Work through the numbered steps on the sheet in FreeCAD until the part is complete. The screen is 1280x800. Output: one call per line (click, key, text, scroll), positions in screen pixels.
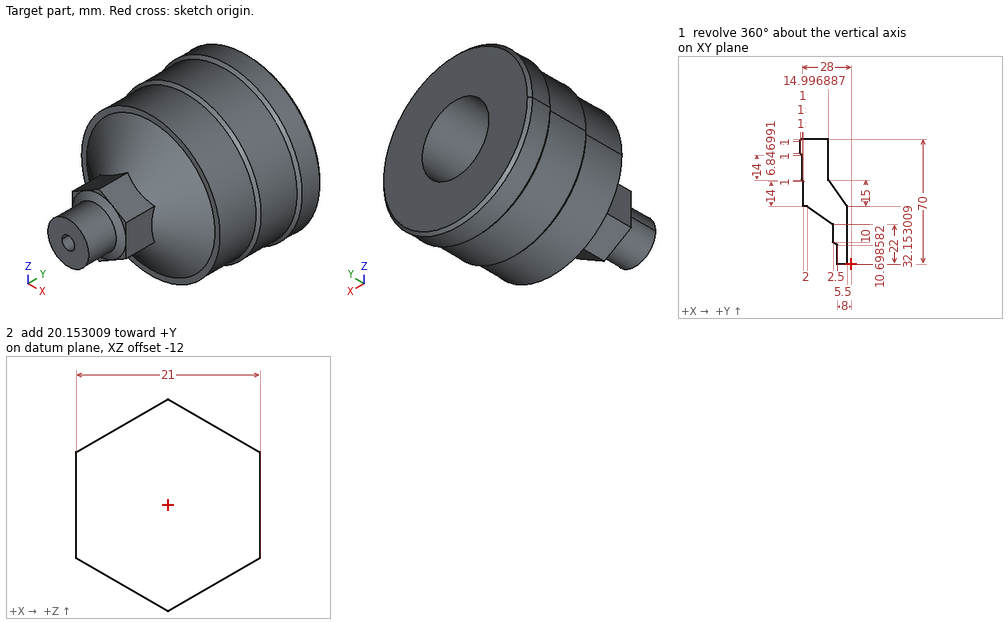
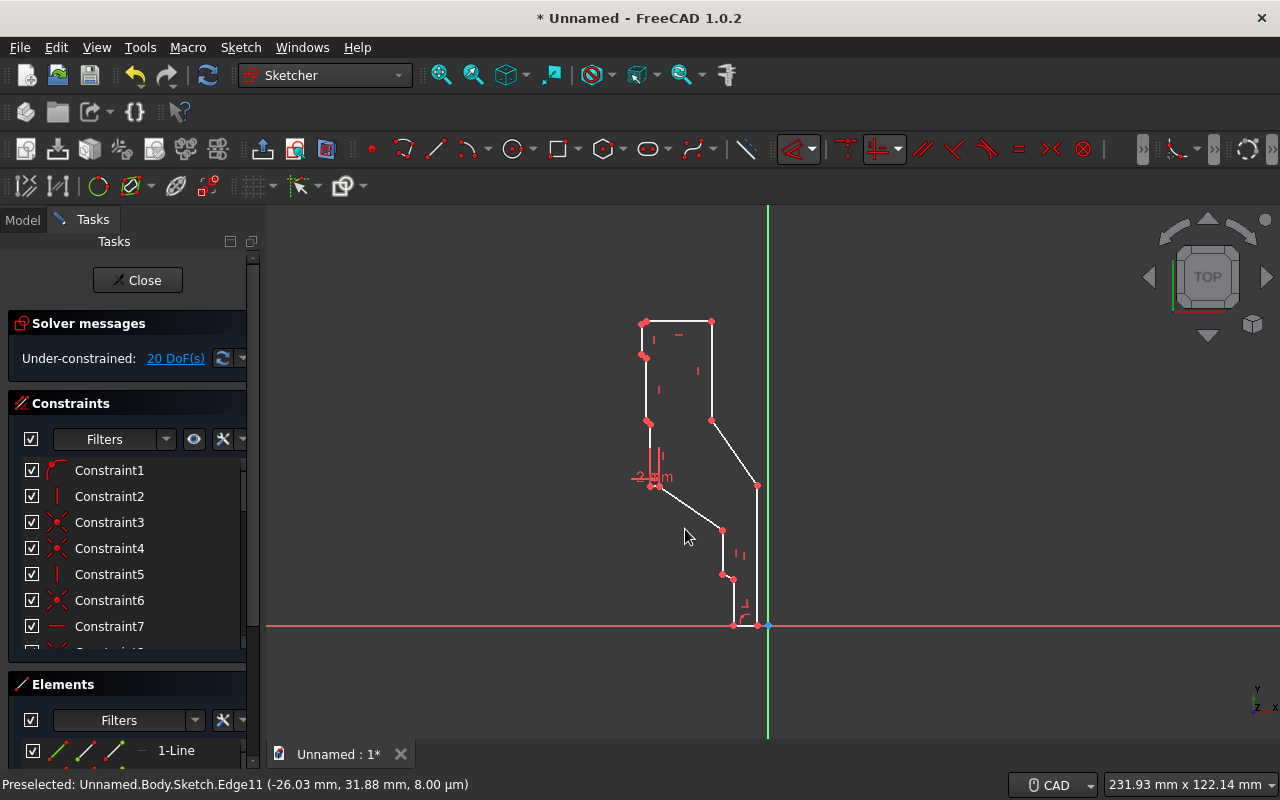
click(646, 377)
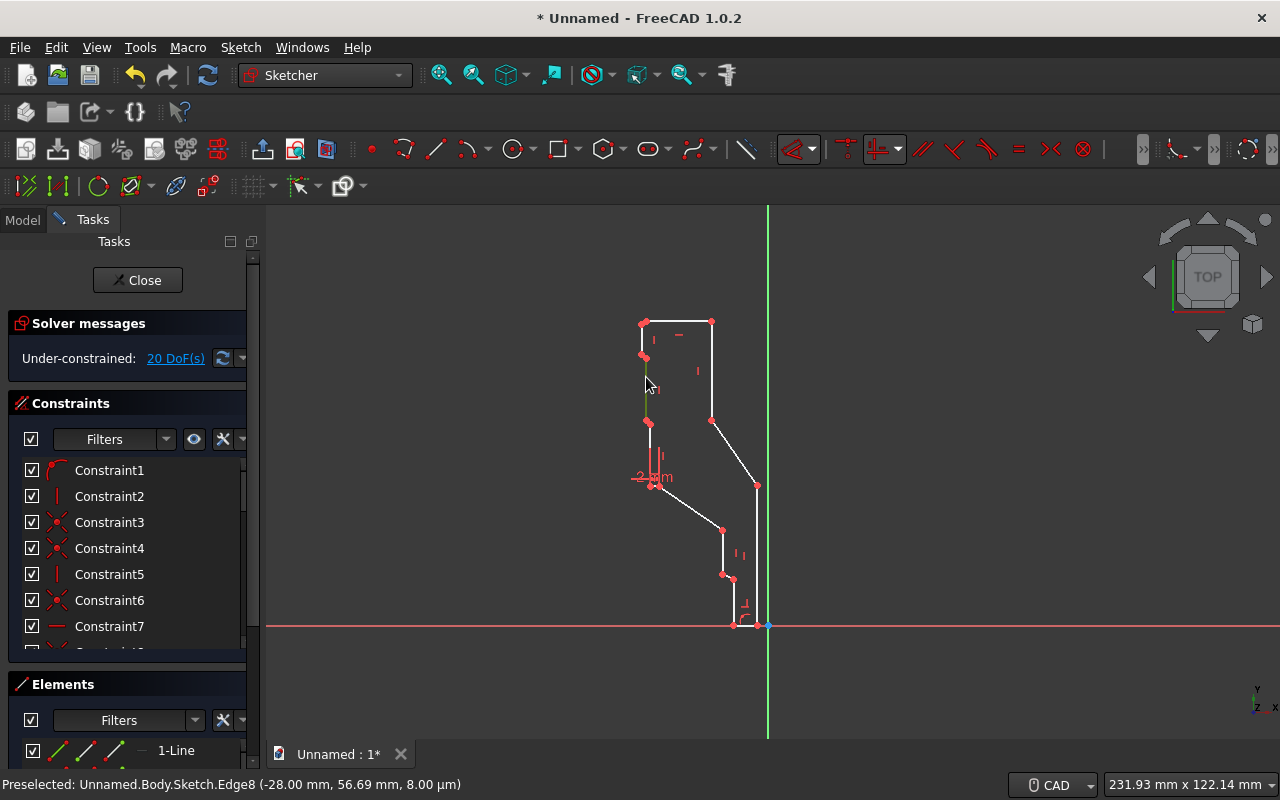
key(i)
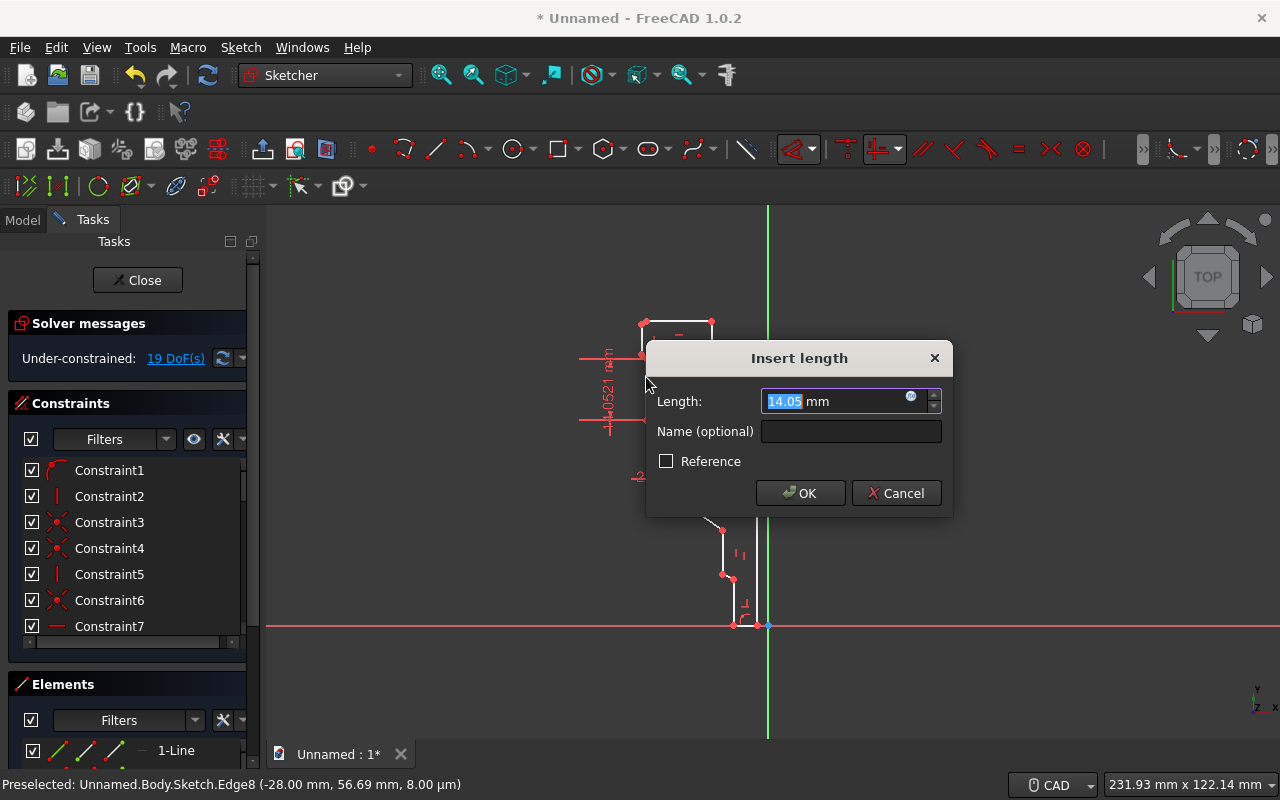
text(14)
key(Return)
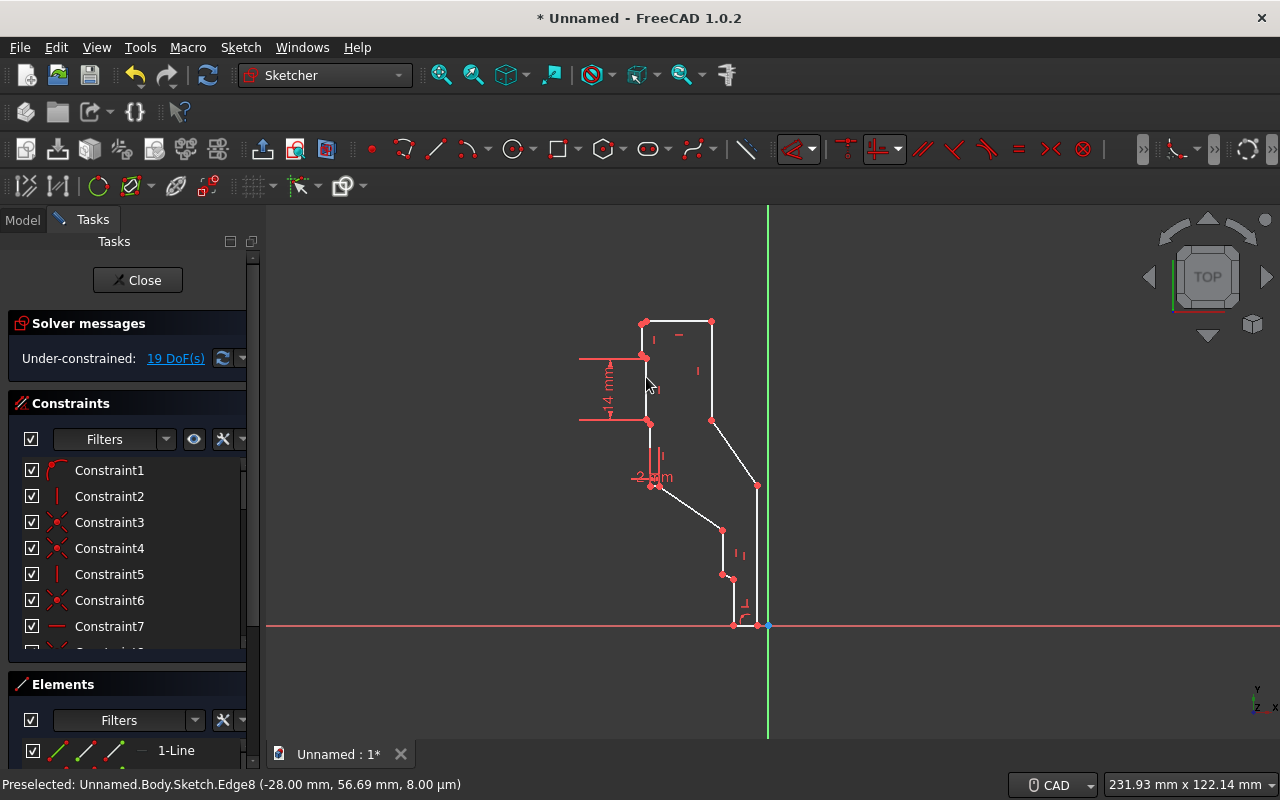
click(650, 443)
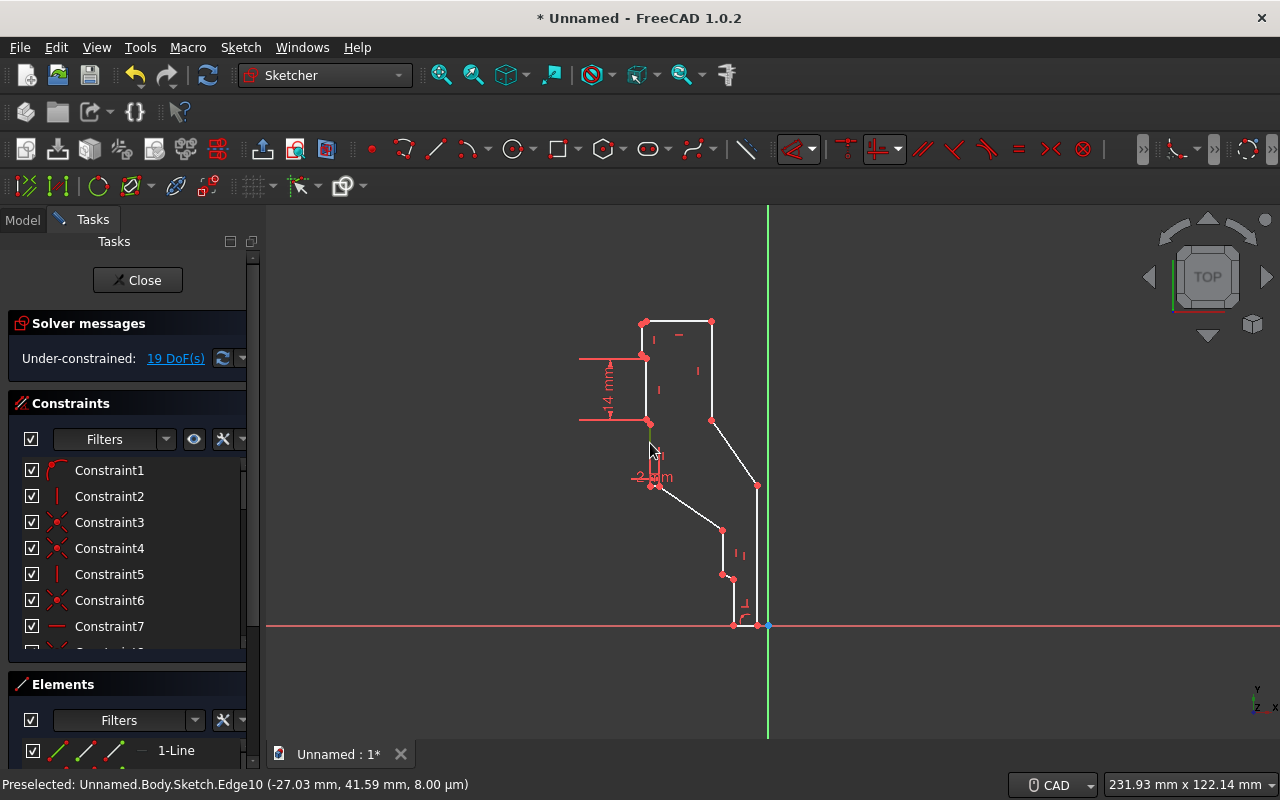
key(i)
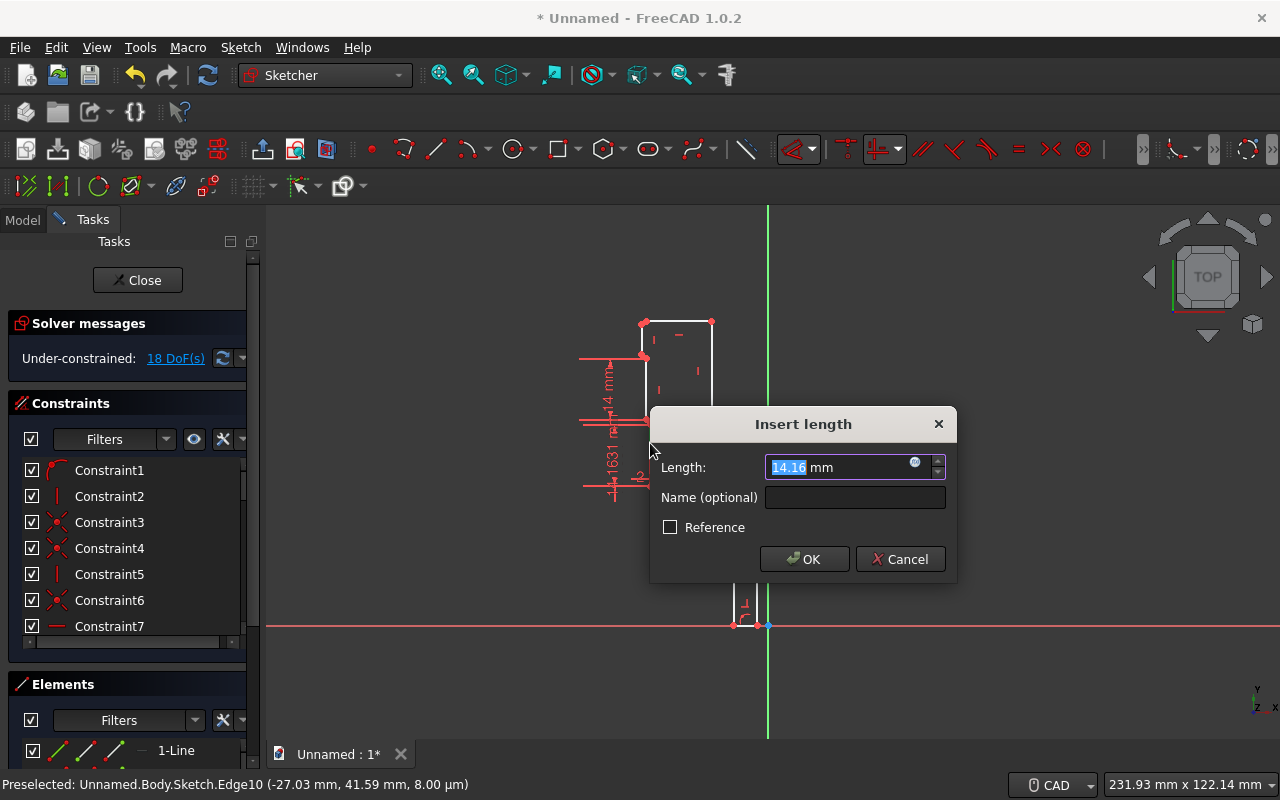
text(14)
key(Return)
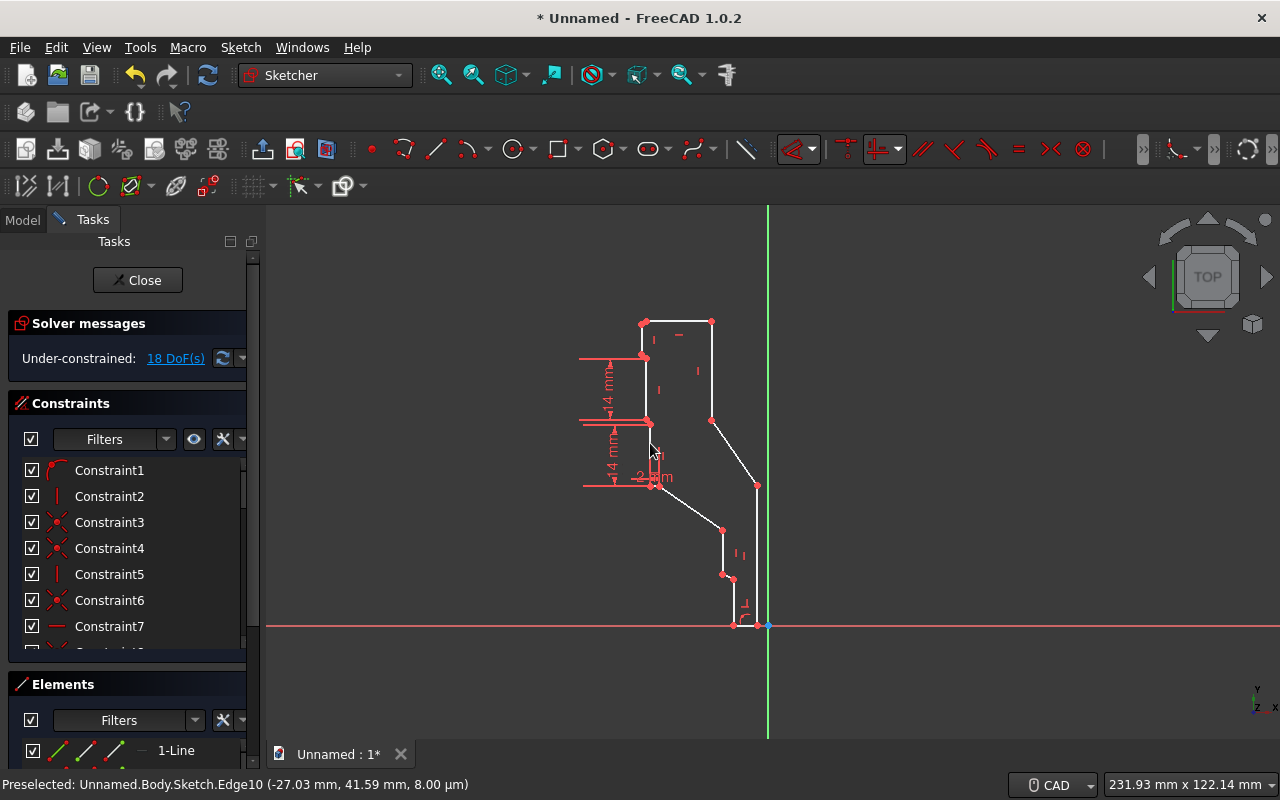
click(723, 543)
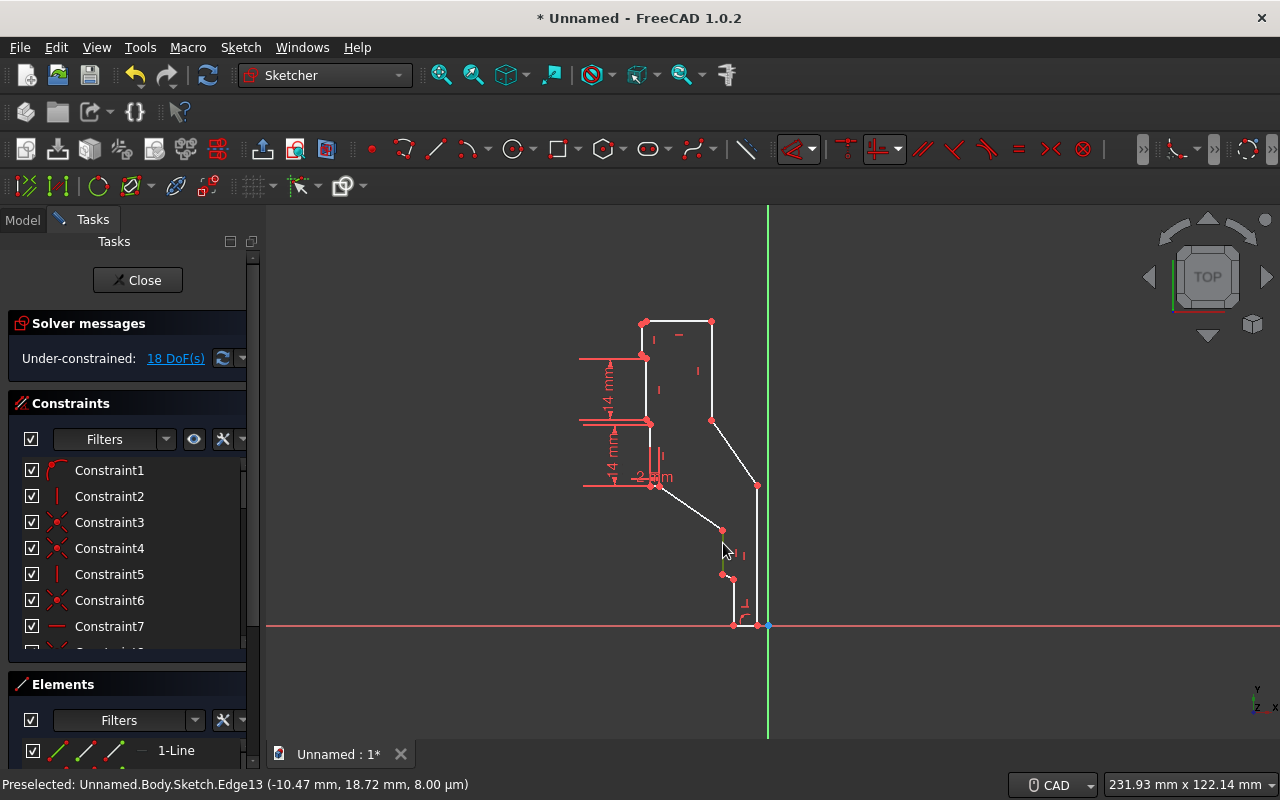
key(i)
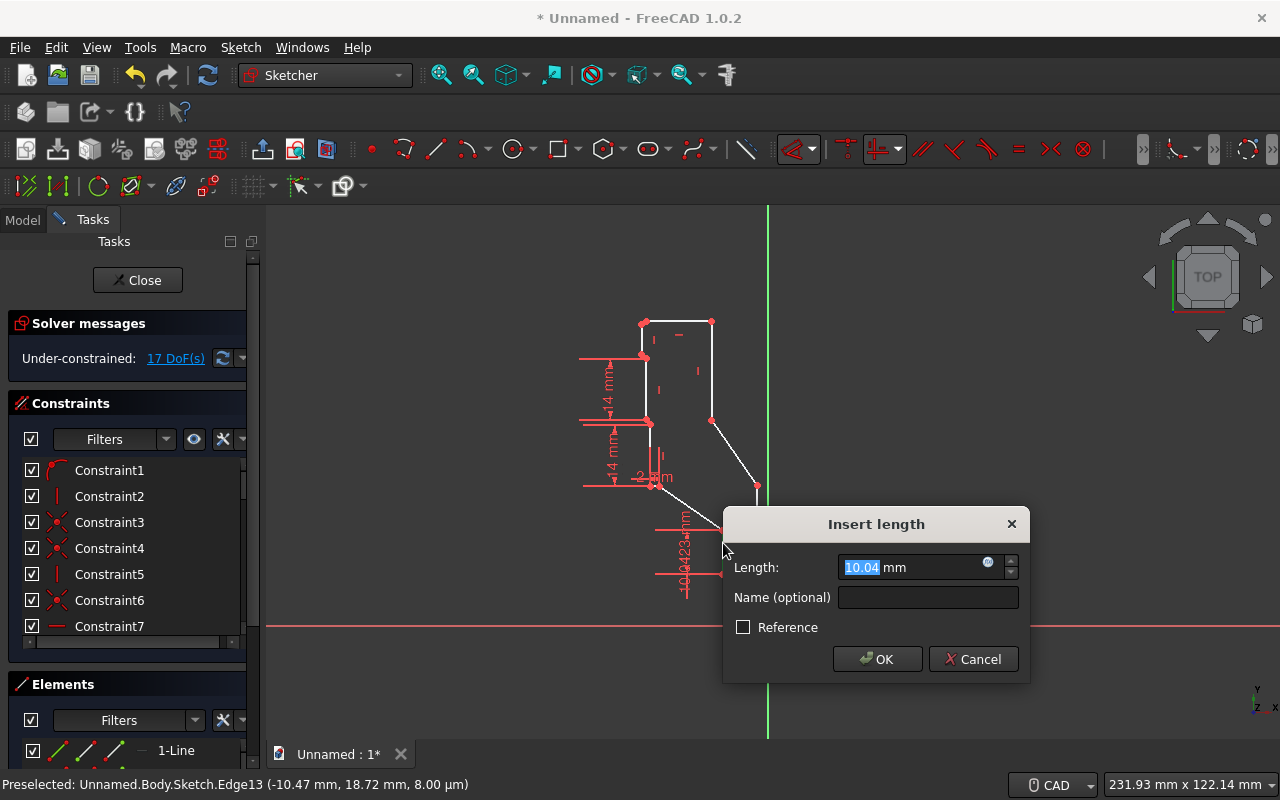
text(10)
key(Return)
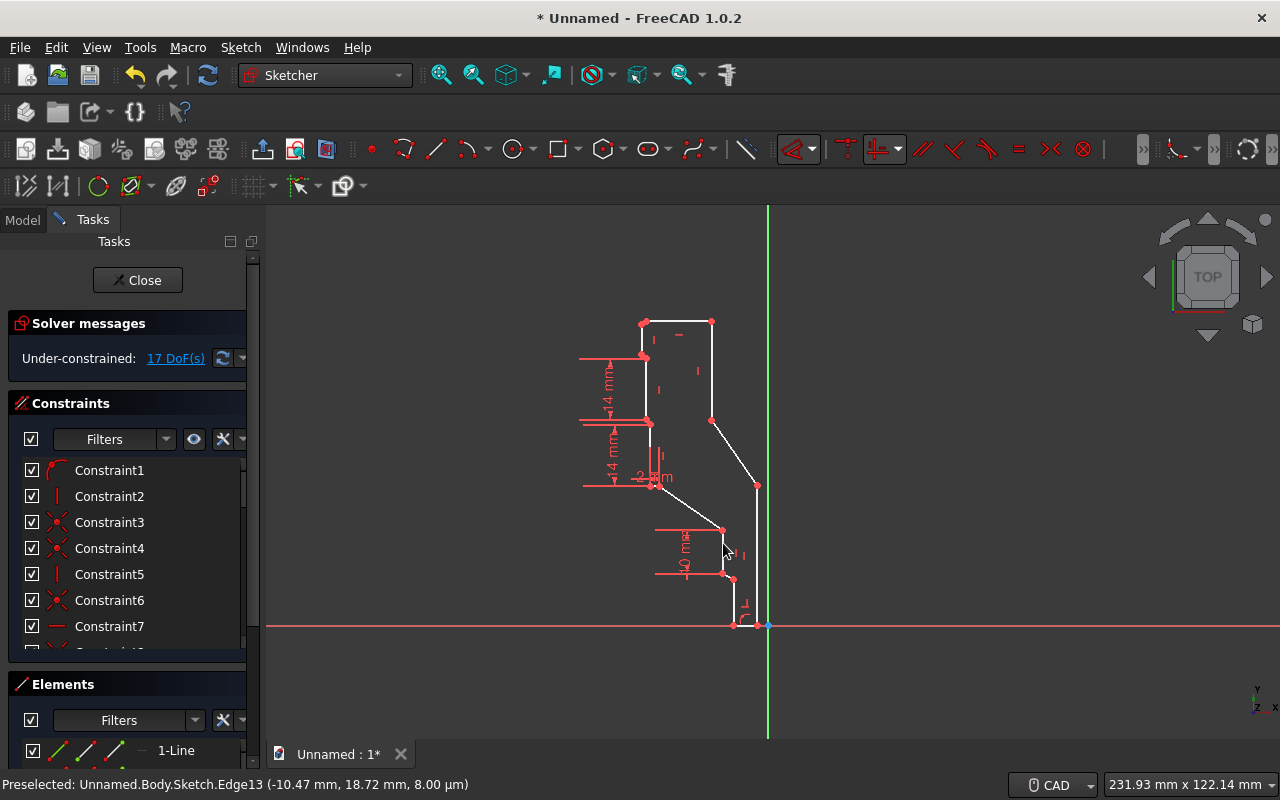
click(734, 580)